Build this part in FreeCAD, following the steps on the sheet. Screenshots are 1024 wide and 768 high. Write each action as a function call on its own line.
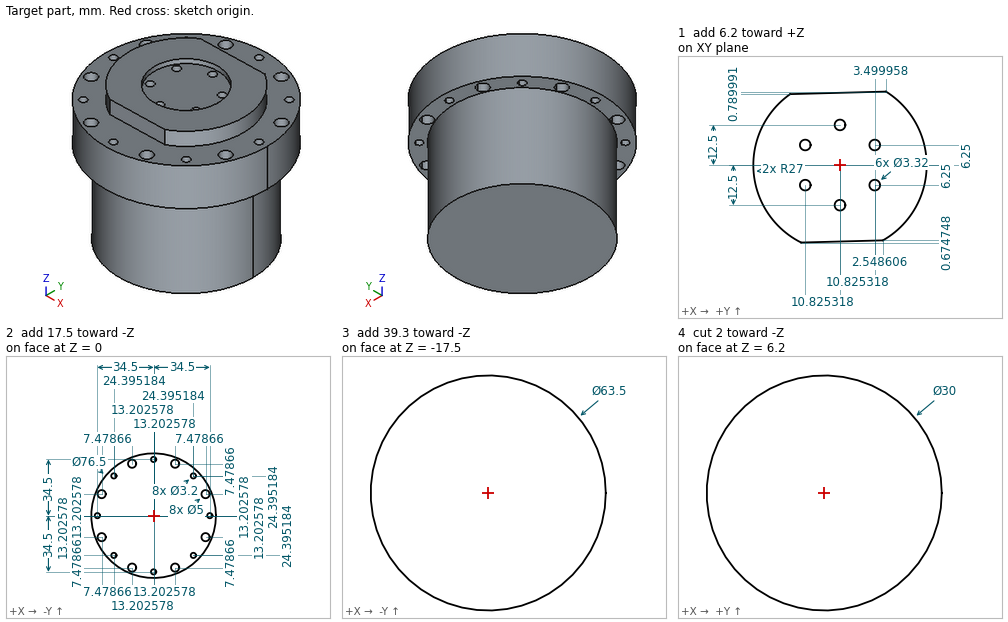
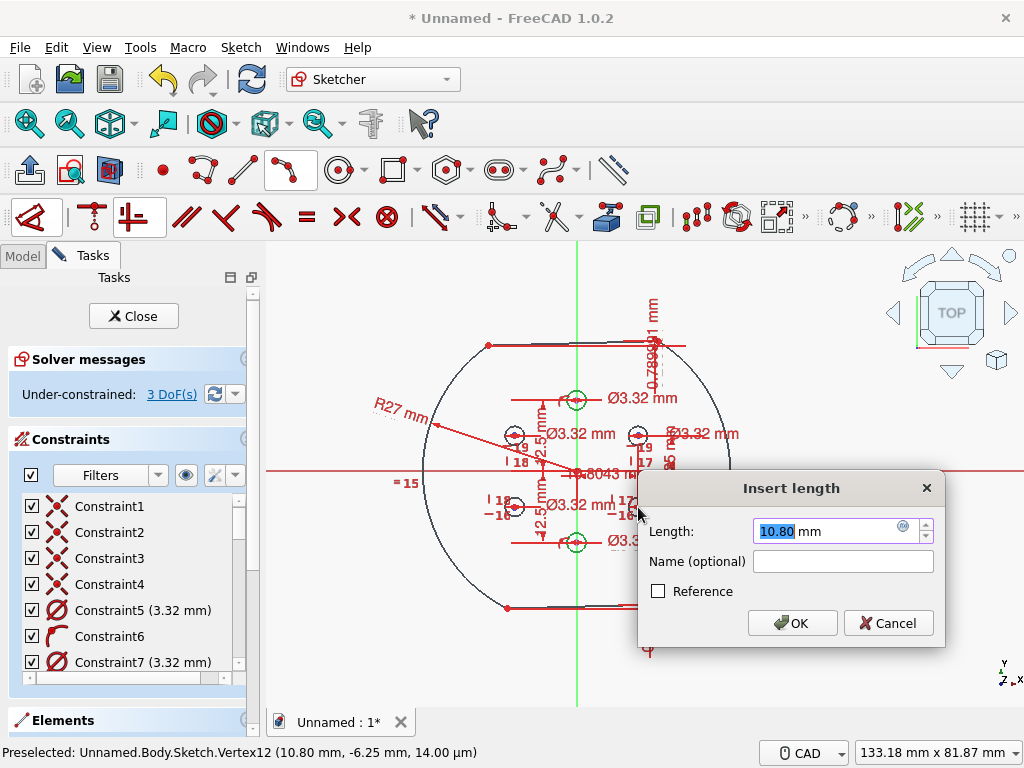
text(10.825318)
key(Return)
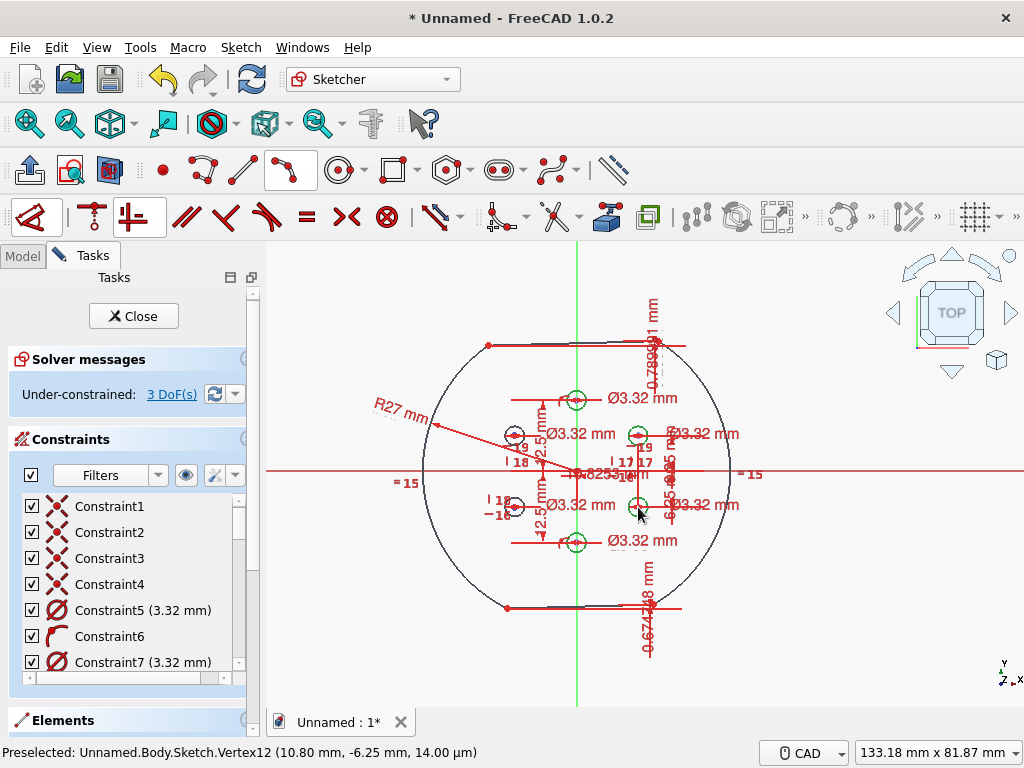
click(515, 507)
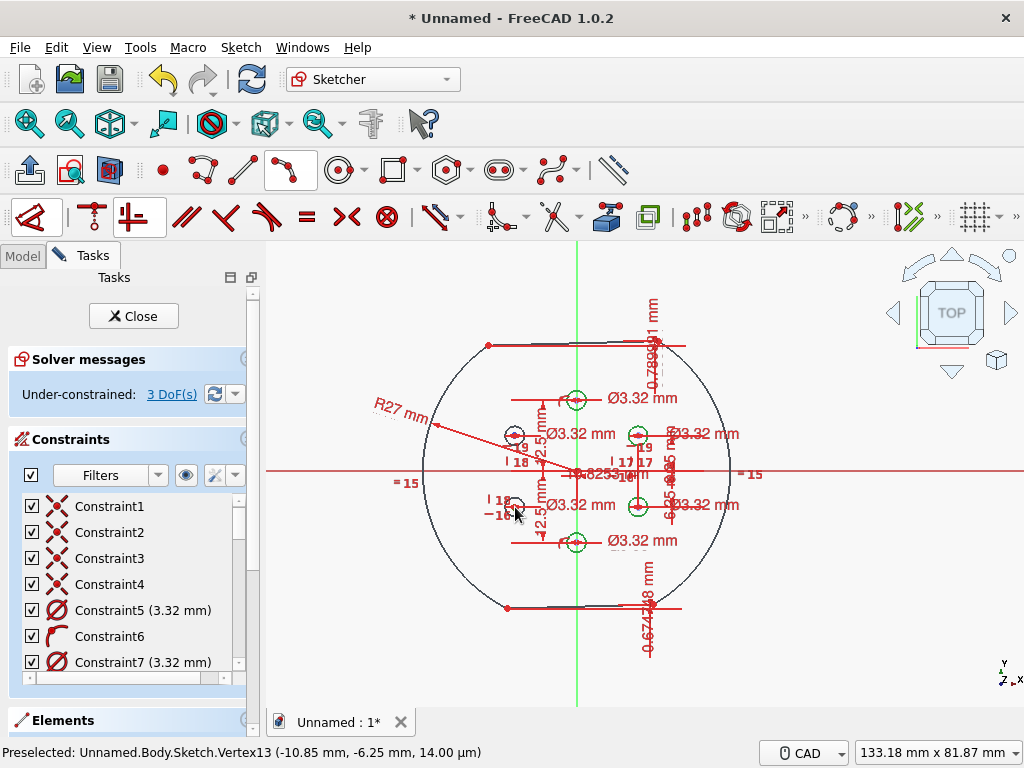
click(56, 218)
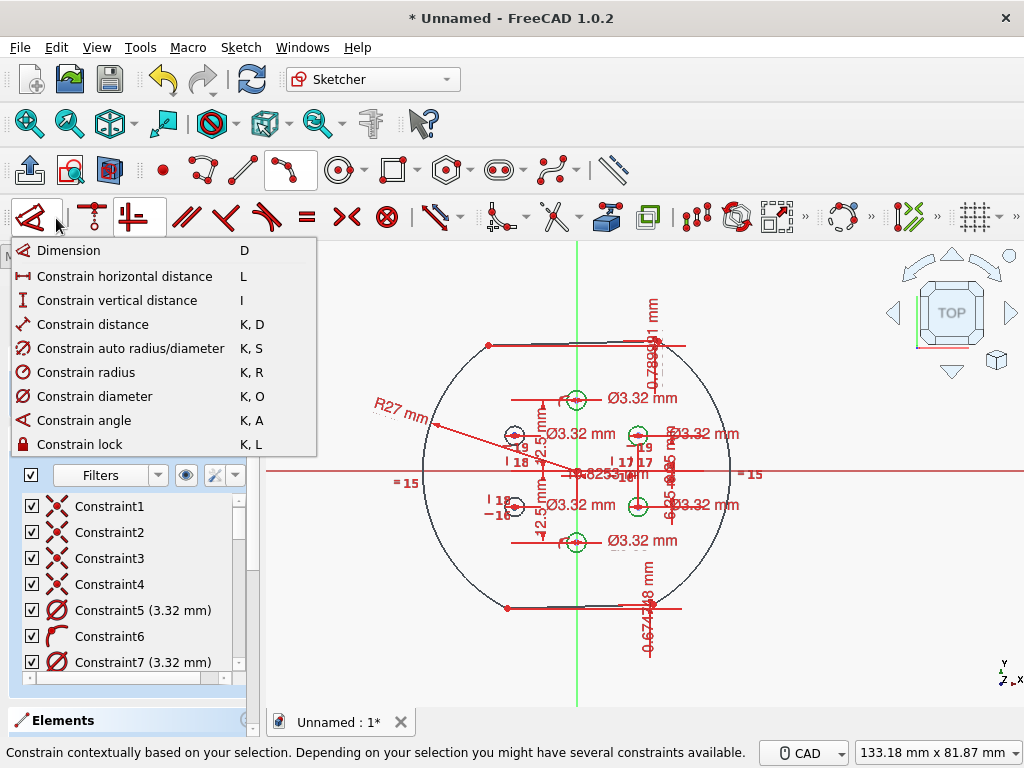
click(164, 276)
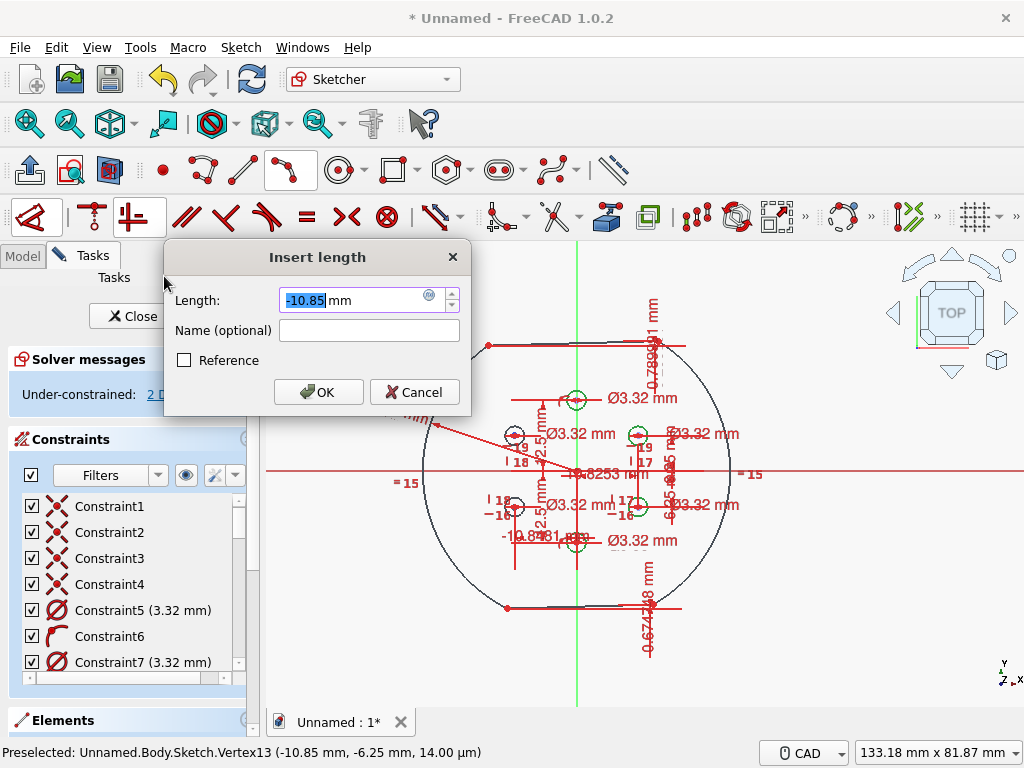
text(-10.825318)
key(Return)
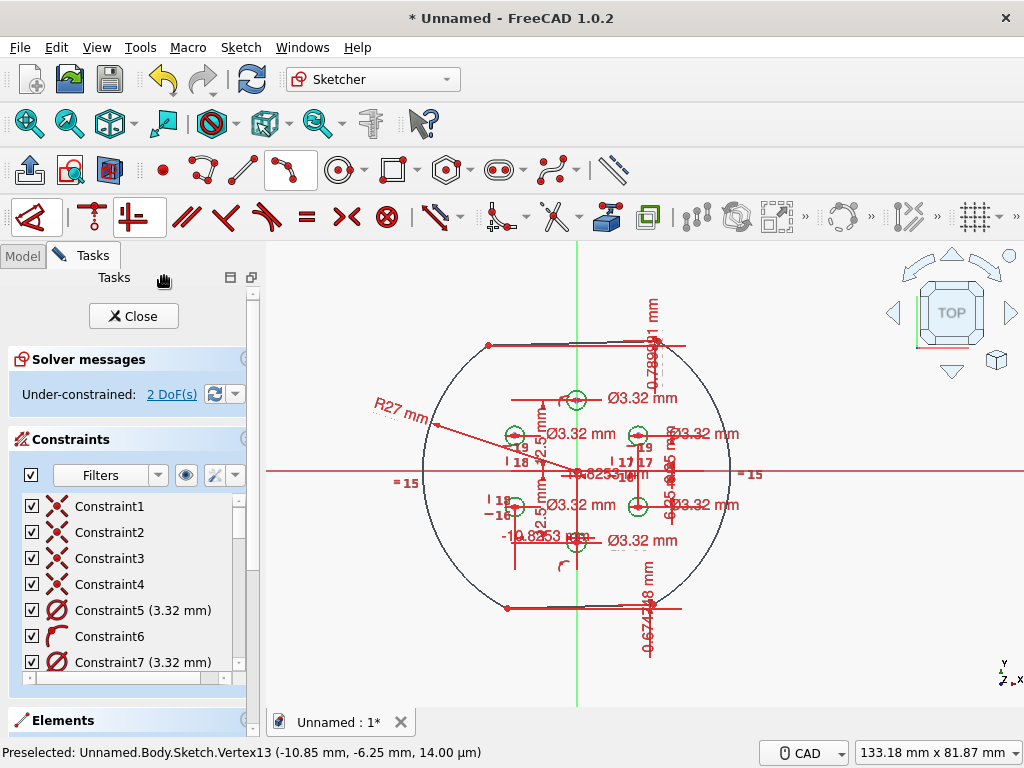
scroll(653, 605, up, 6)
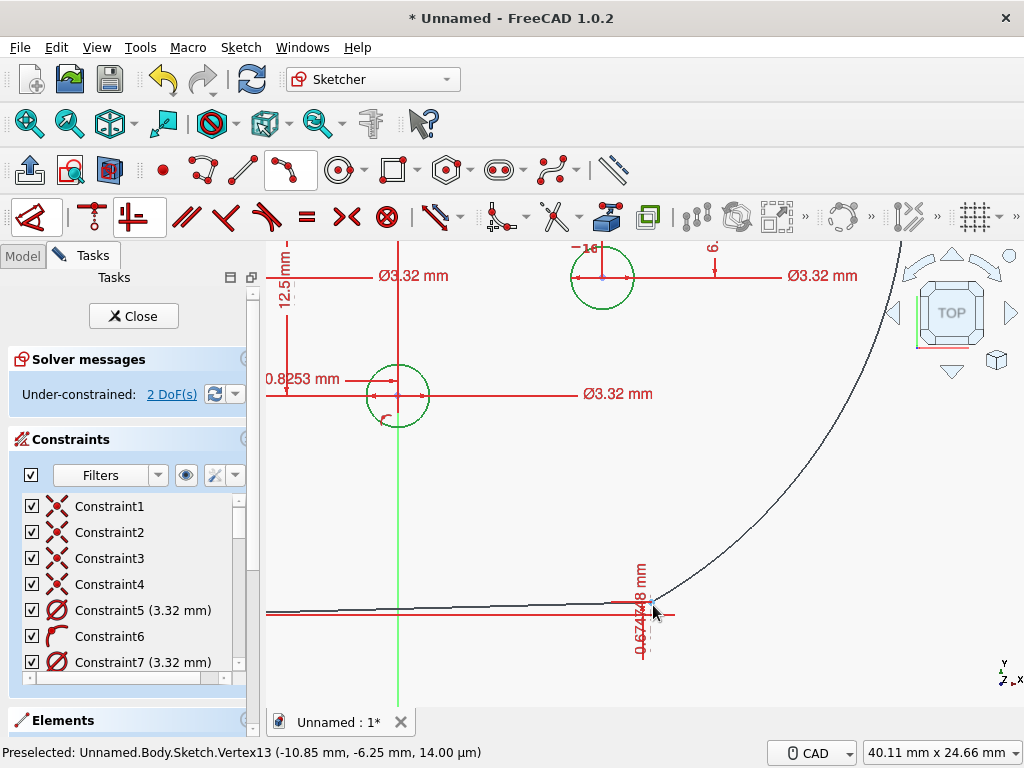
click(652, 602)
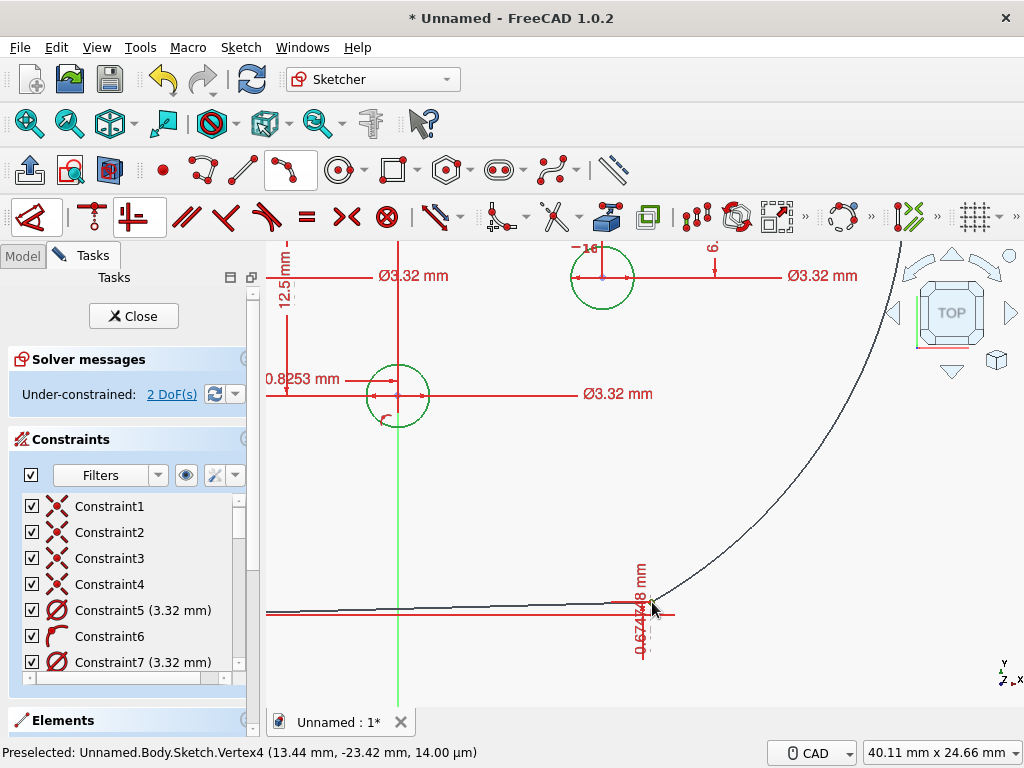
click(602, 278)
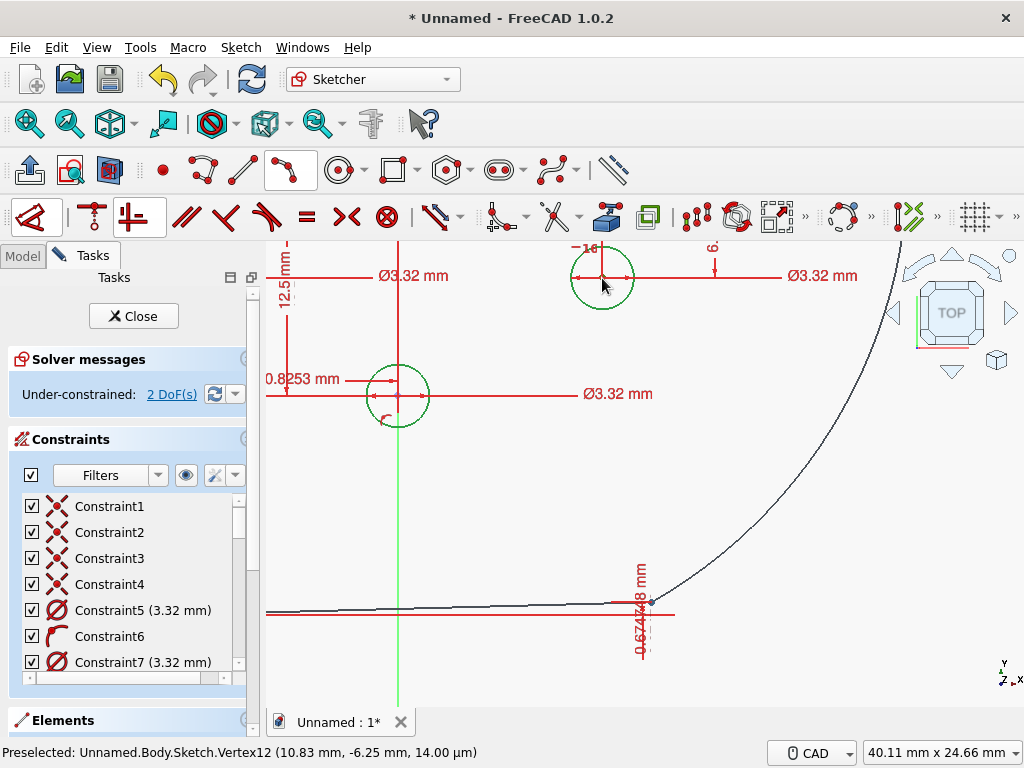
key(l)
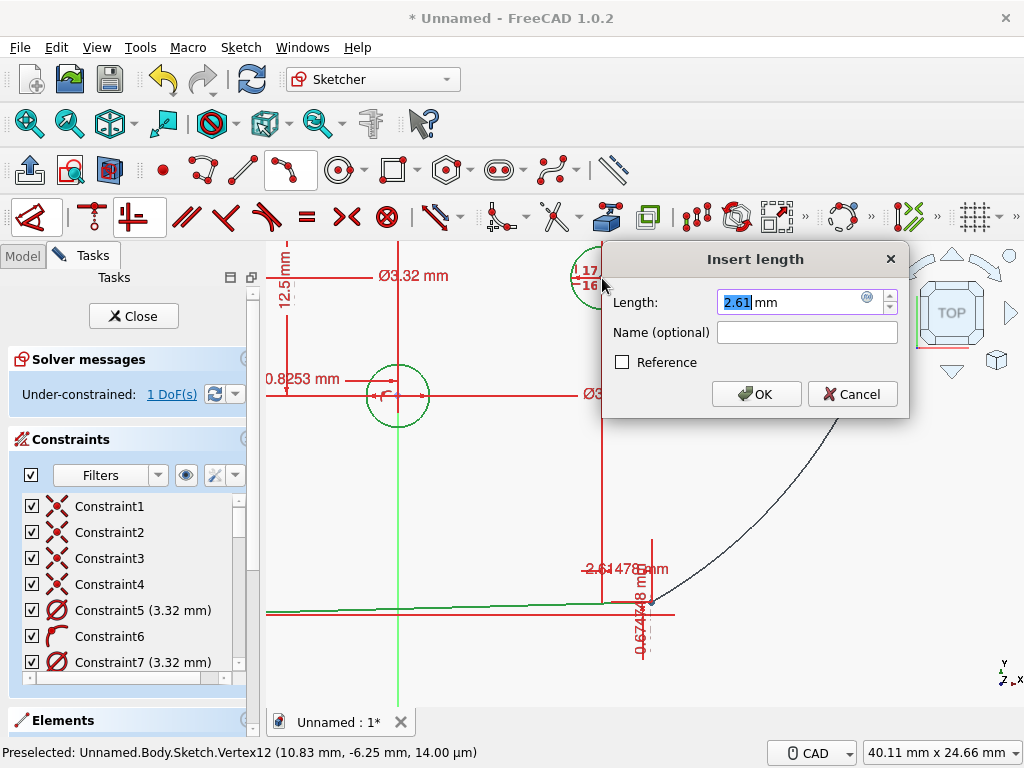
text(2.548606)
key(Return)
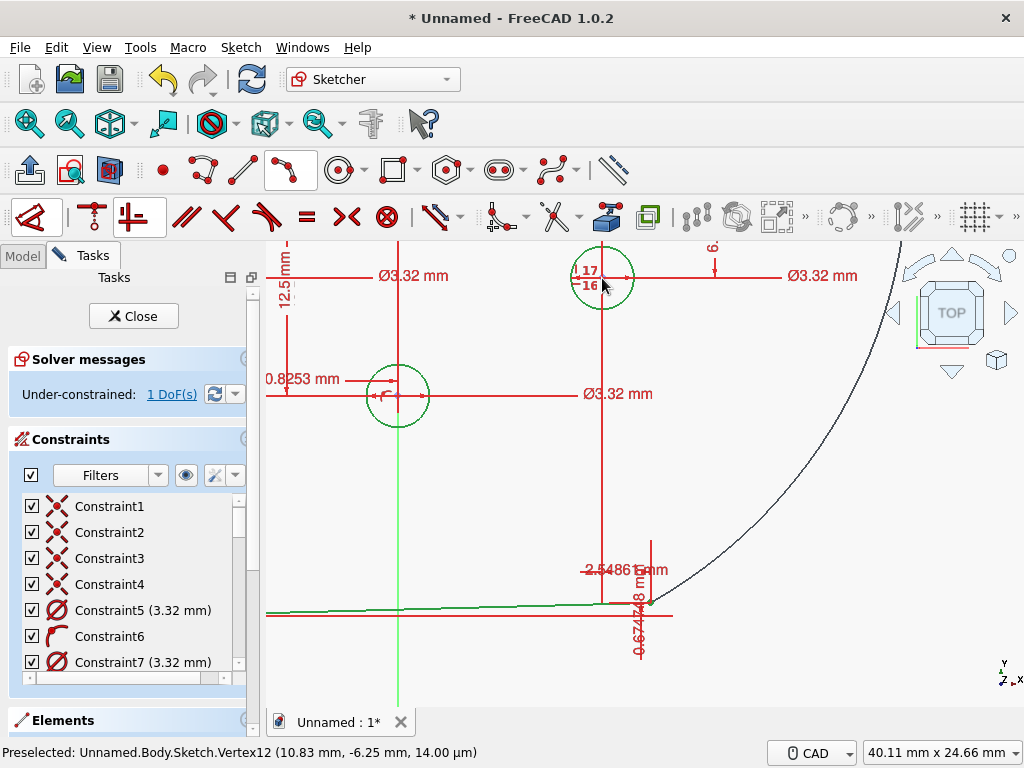
scroll(653, 604, down, 6)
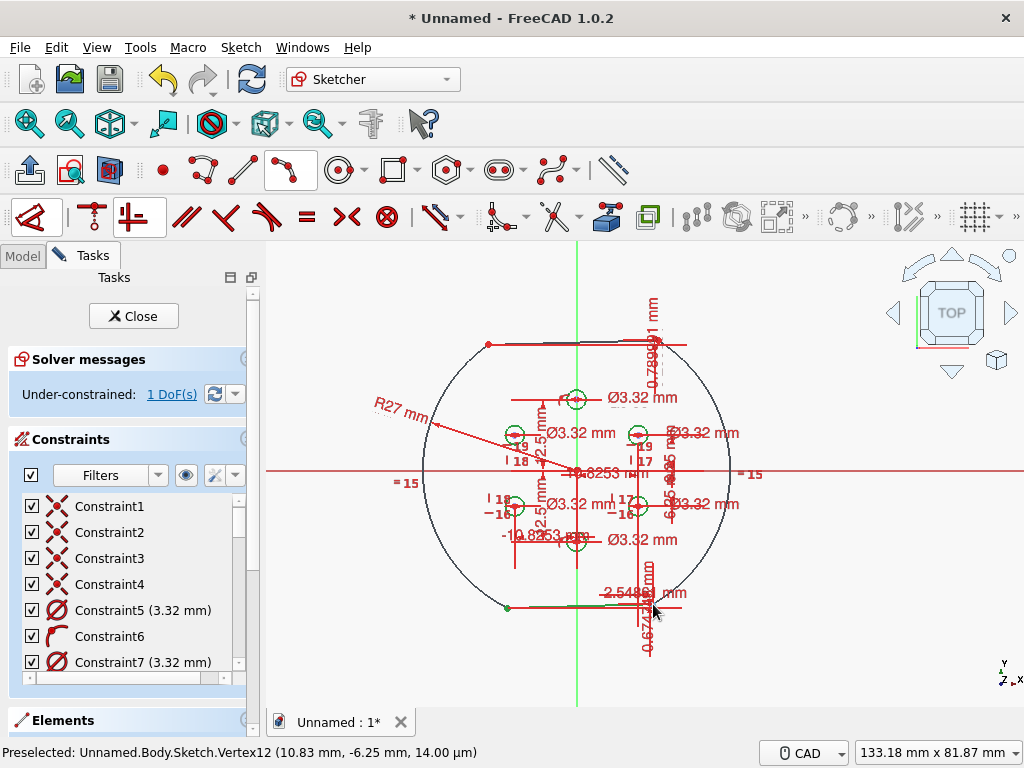
scroll(658, 340, up, 4)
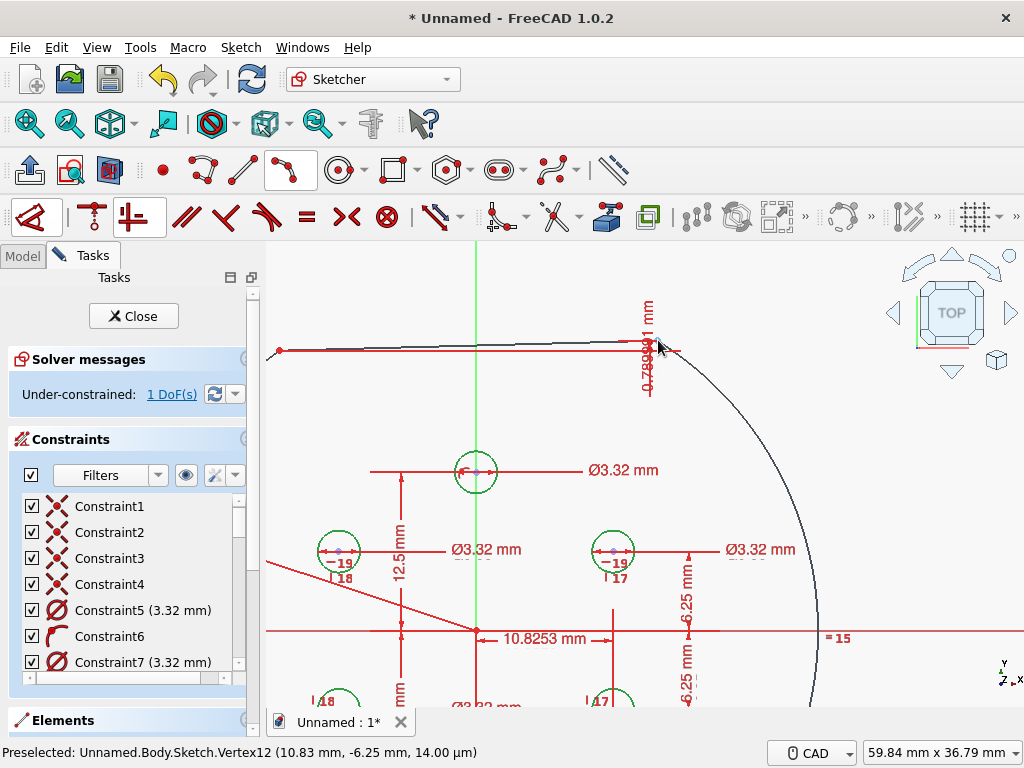
click(657, 341)